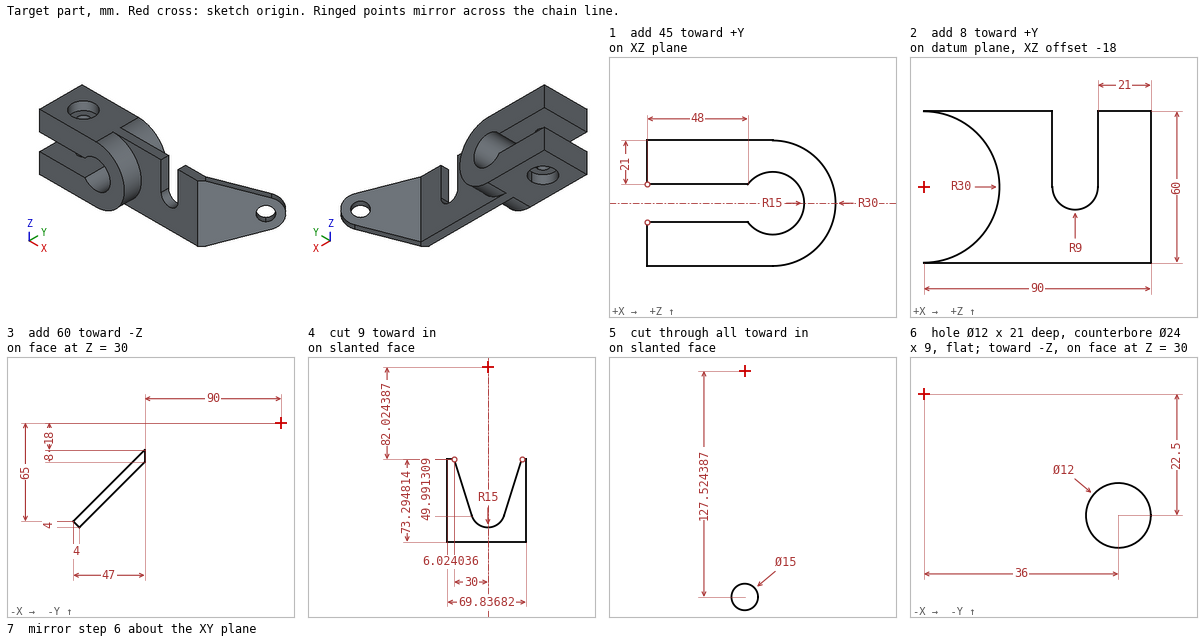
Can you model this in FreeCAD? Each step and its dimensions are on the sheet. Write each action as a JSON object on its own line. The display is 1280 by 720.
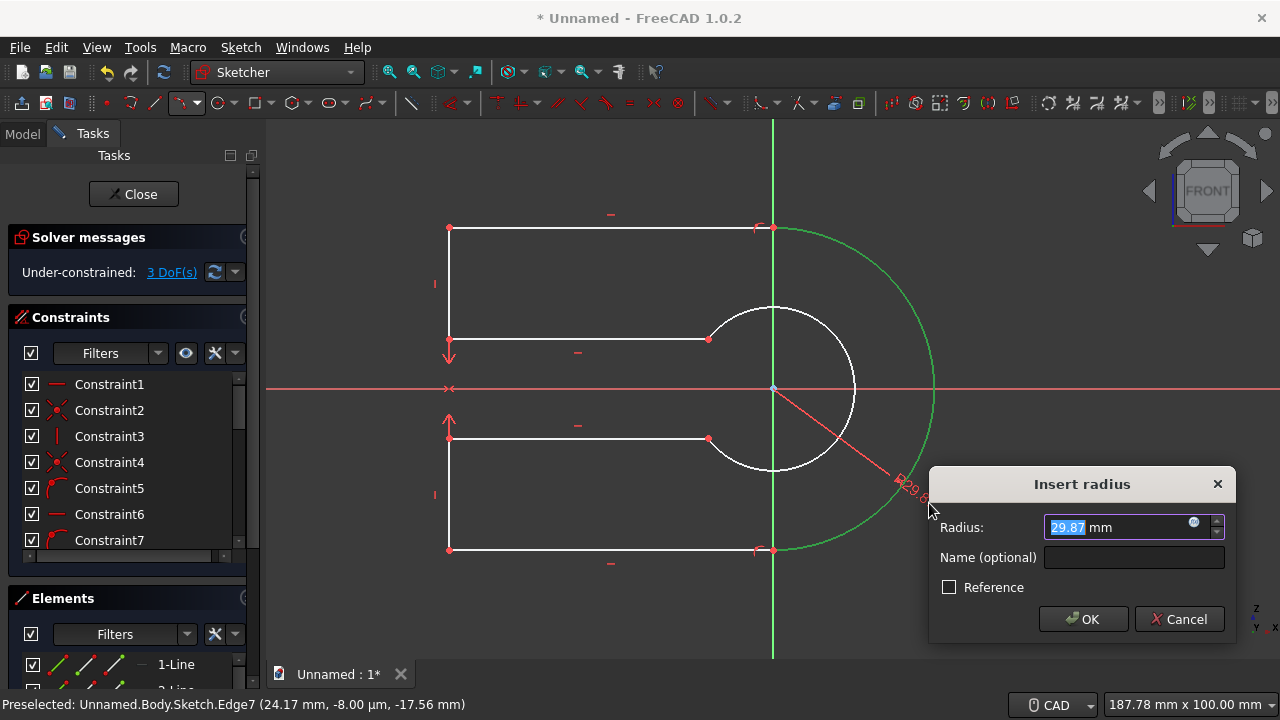
{"action": "type", "text": "30"}
{"action": "key", "text": "Return"}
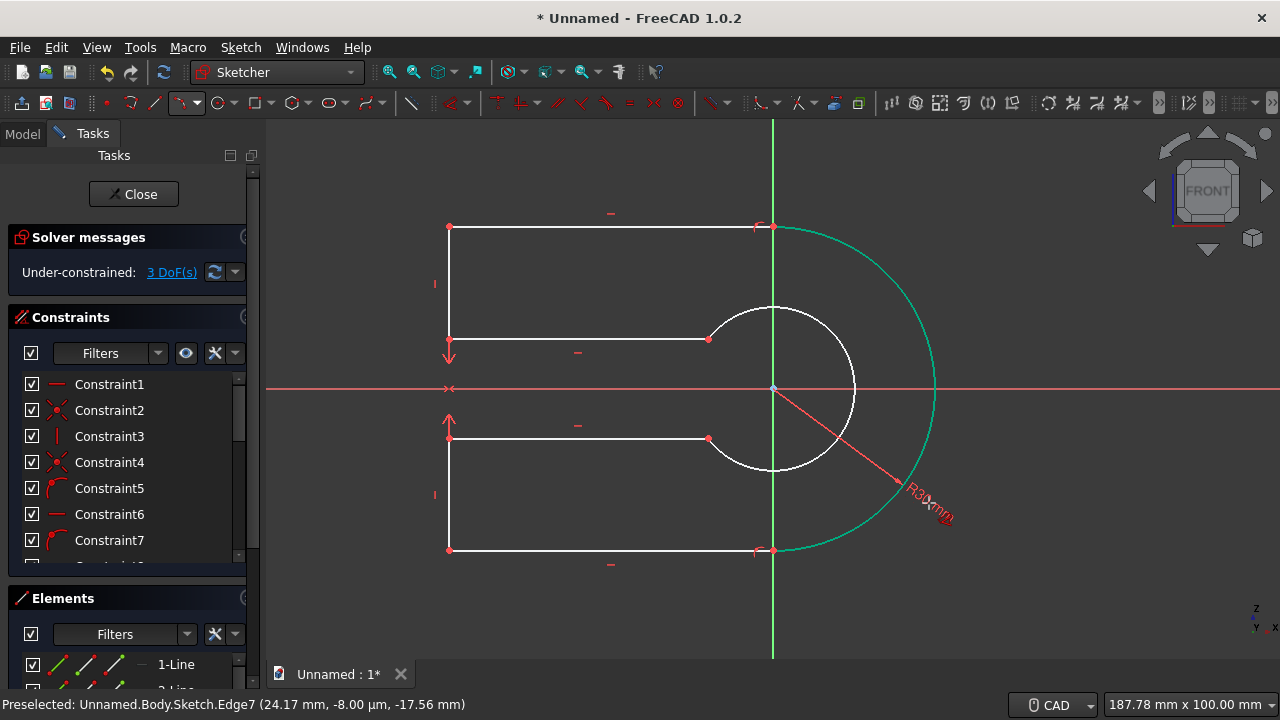
{"action": "left_click", "coordinate": [818, 458]}
{"action": "left_click", "coordinate": [835, 485]}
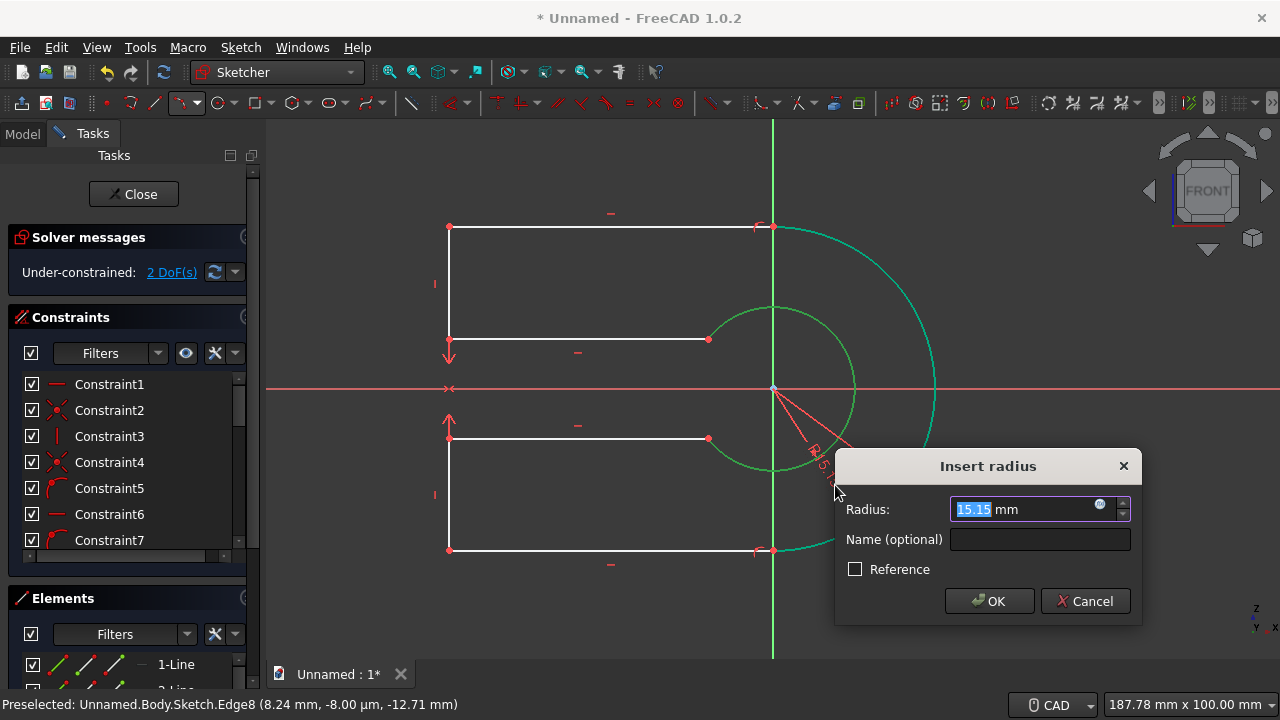
{"action": "type", "text": "15"}
{"action": "key", "text": "Return"}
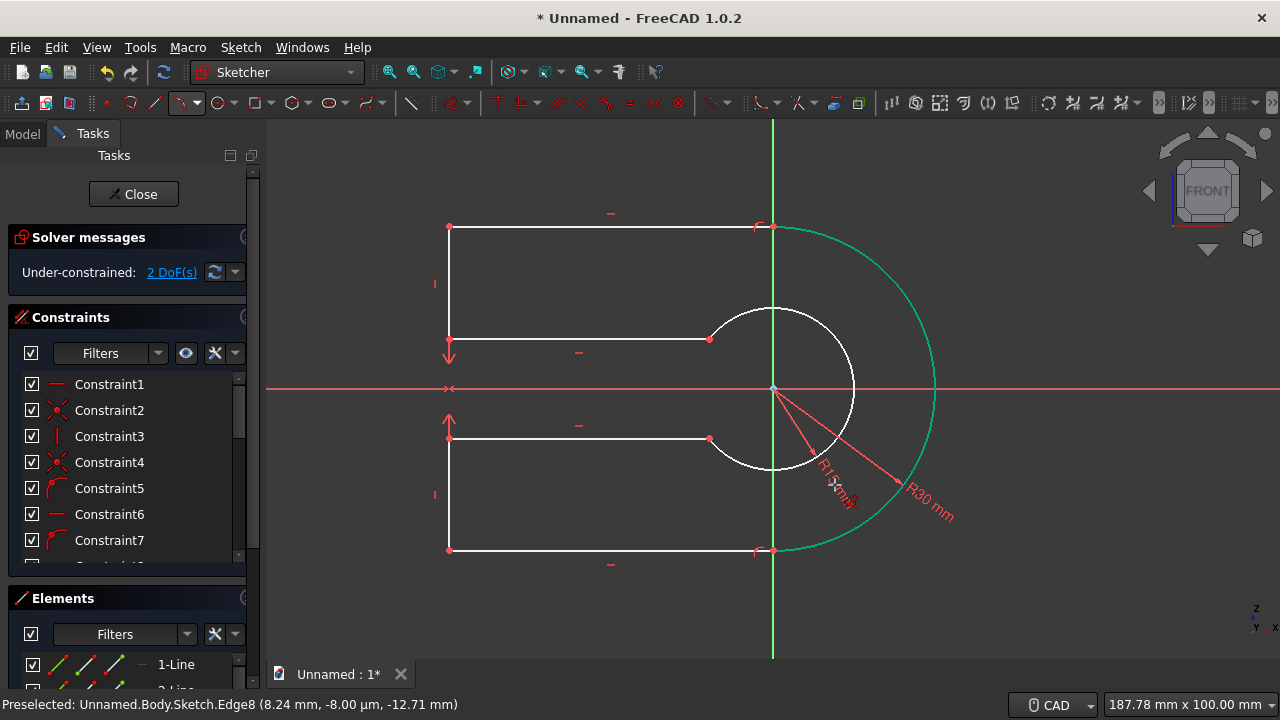
{"action": "left_click", "coordinate": [631, 339]}
{"action": "left_click", "coordinate": [579, 305]}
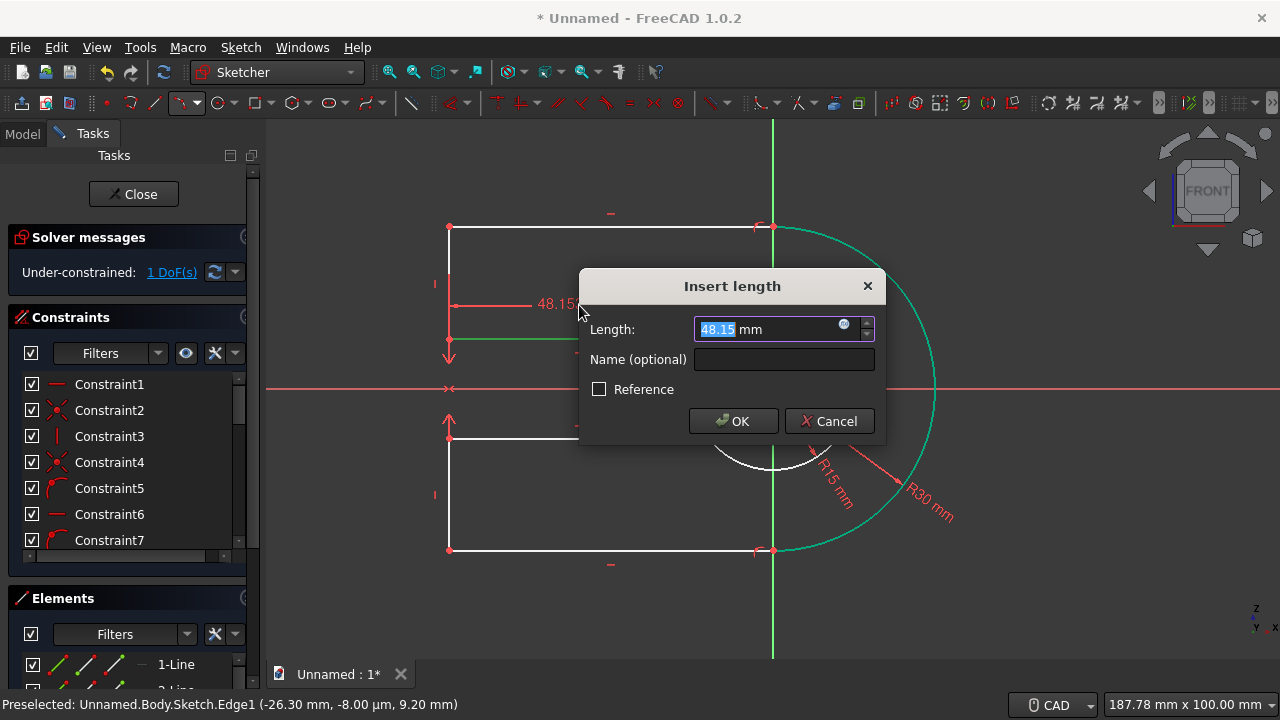
{"action": "type", "text": "48"}
{"action": "key", "text": "Return"}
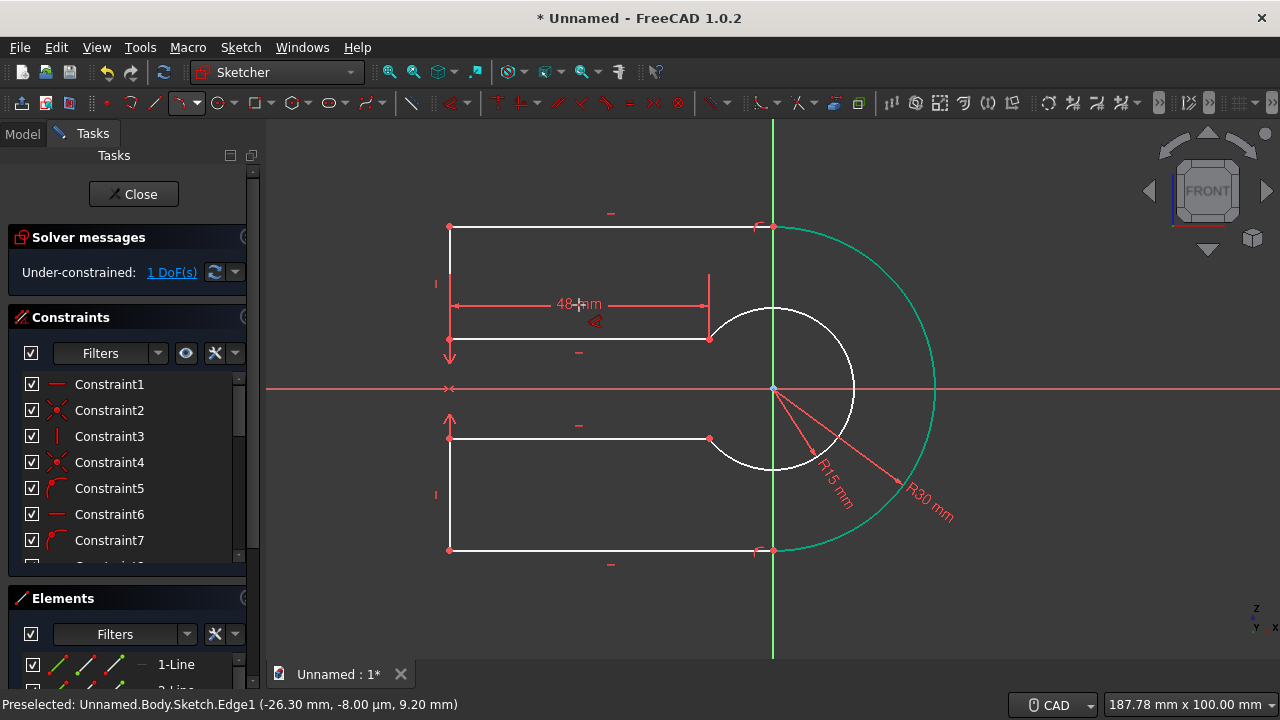
{"action": "left_click", "coordinate": [450, 306]}
{"action": "left_click", "coordinate": [416, 283]}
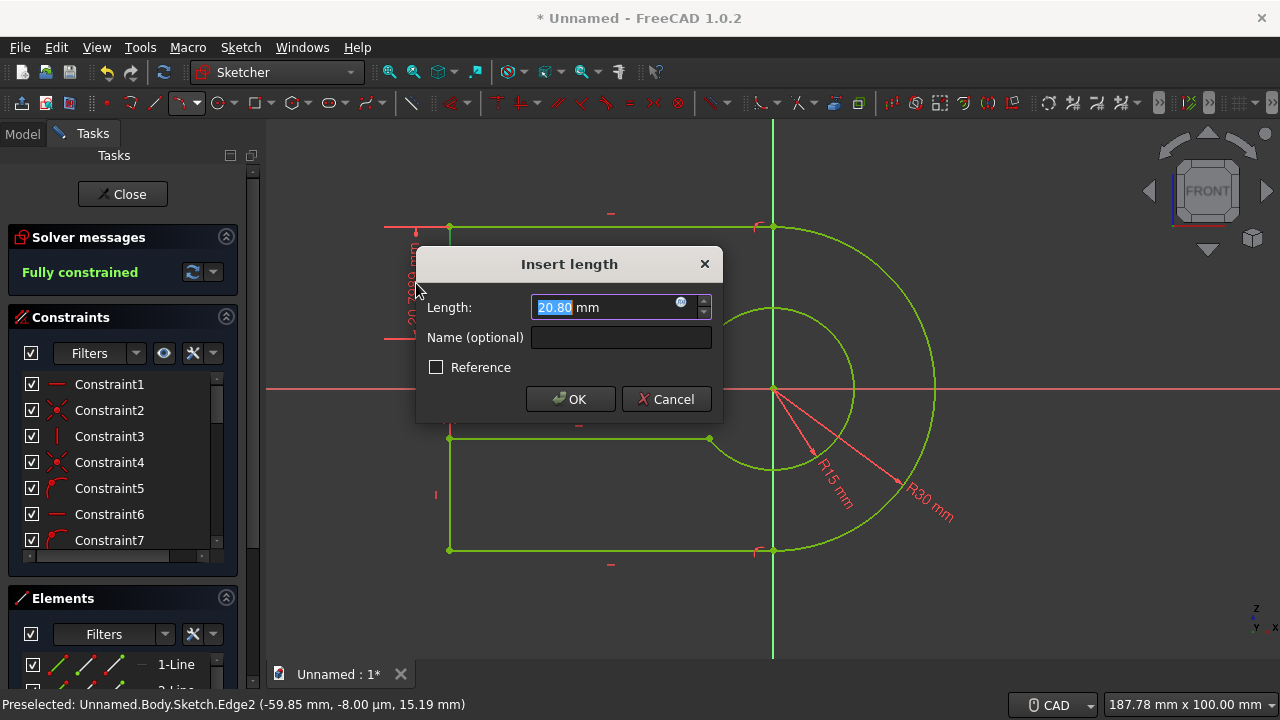
{"action": "type", "text": "21"}
{"action": "key", "text": "Return"}
{"action": "key", "text": "Escape"}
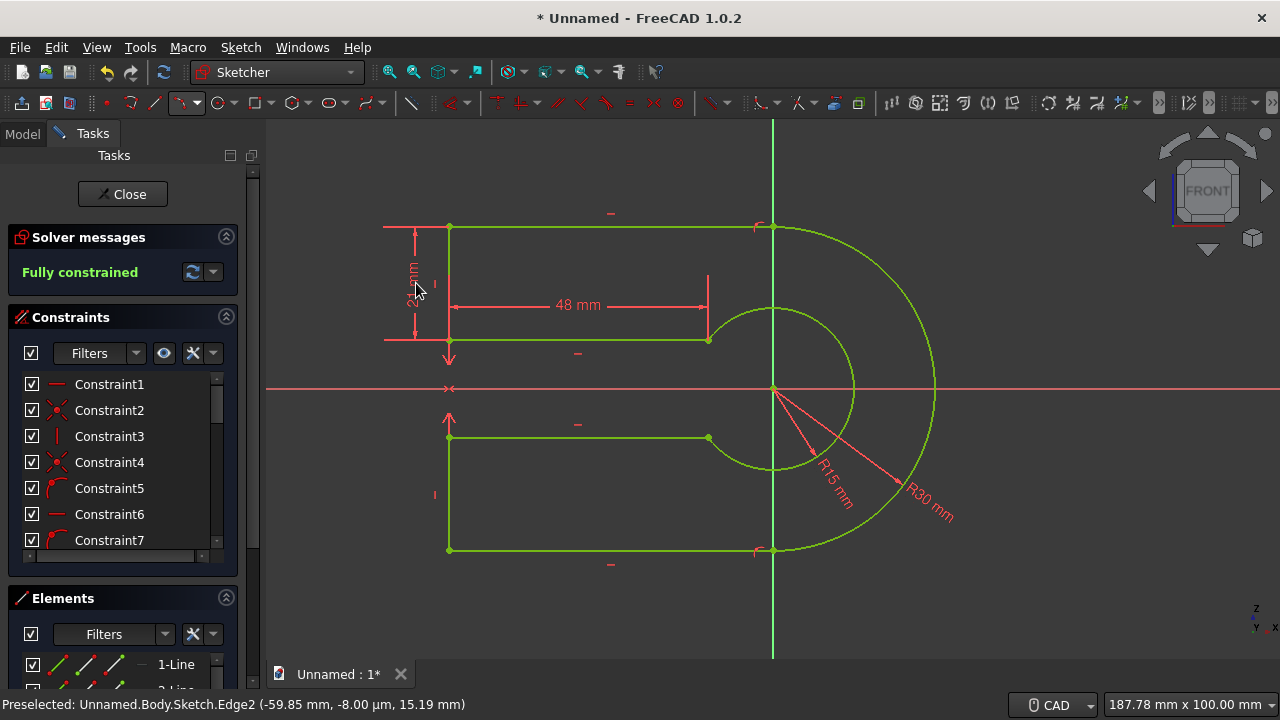
{"action": "left_click", "coordinate": [123, 194]}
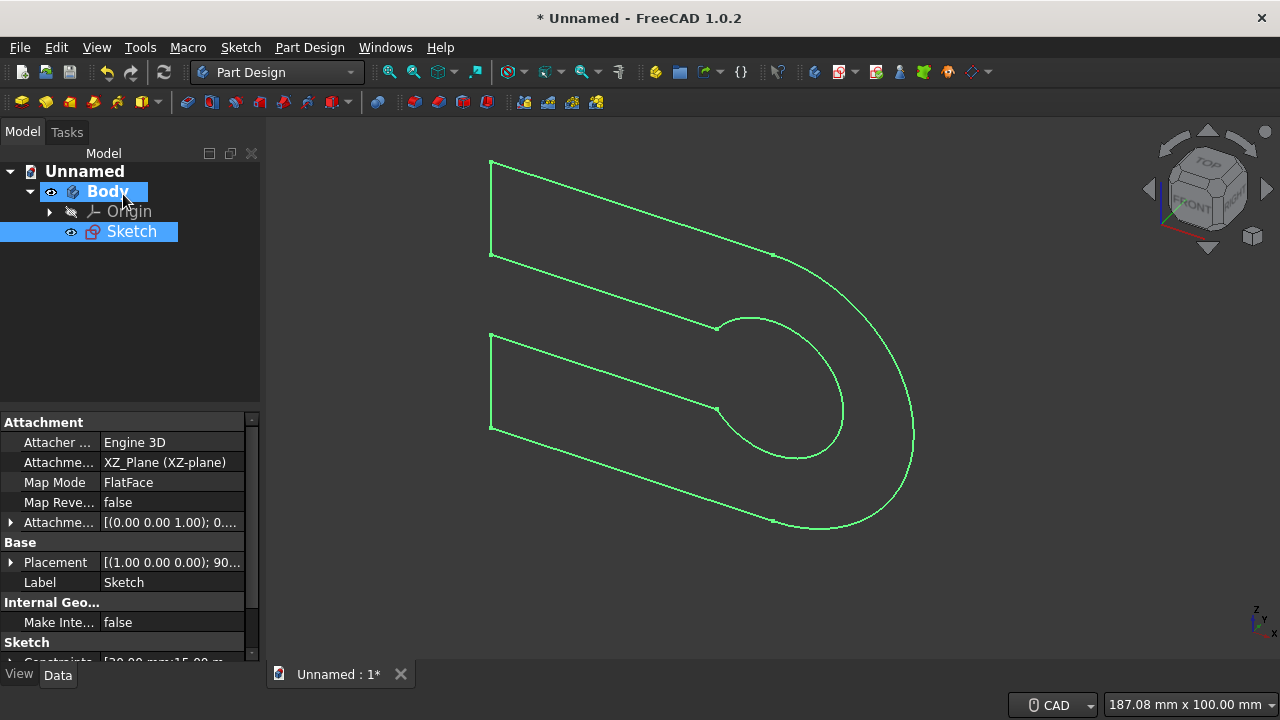
{"action": "left_click", "coordinate": [22, 102]}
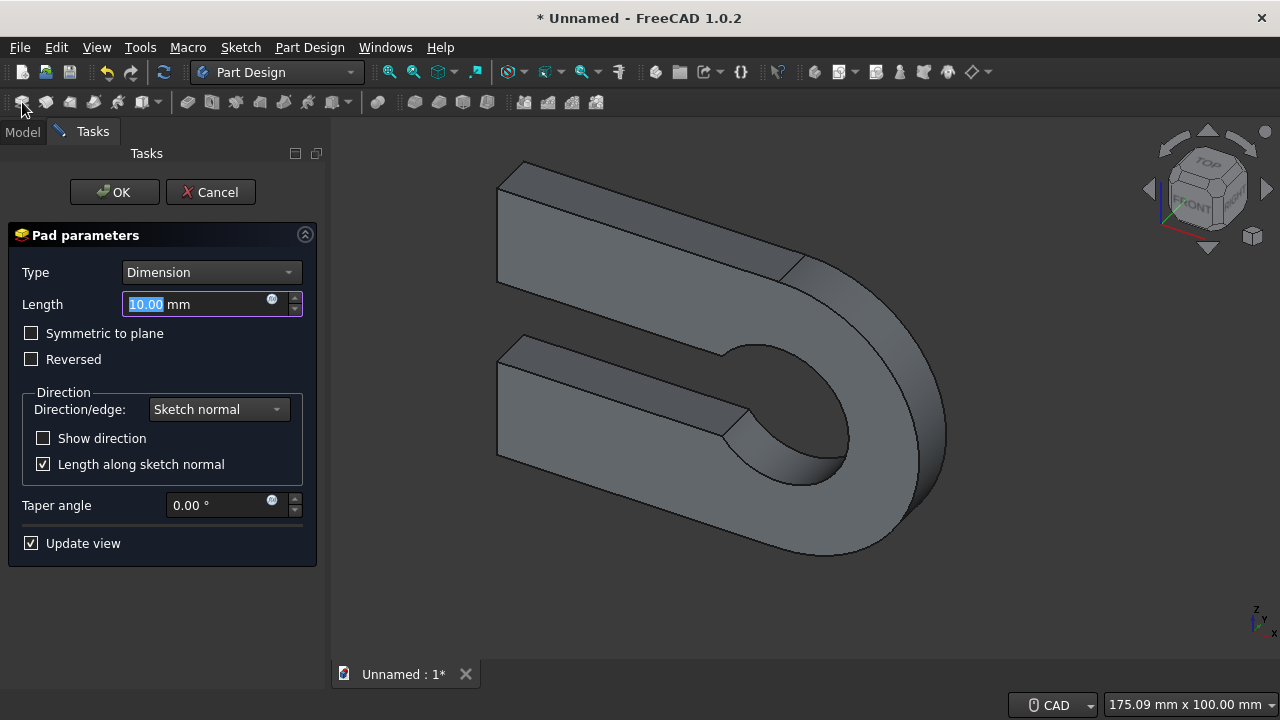
{"action": "type", "text": "45"}
{"action": "key", "text": "Tab"}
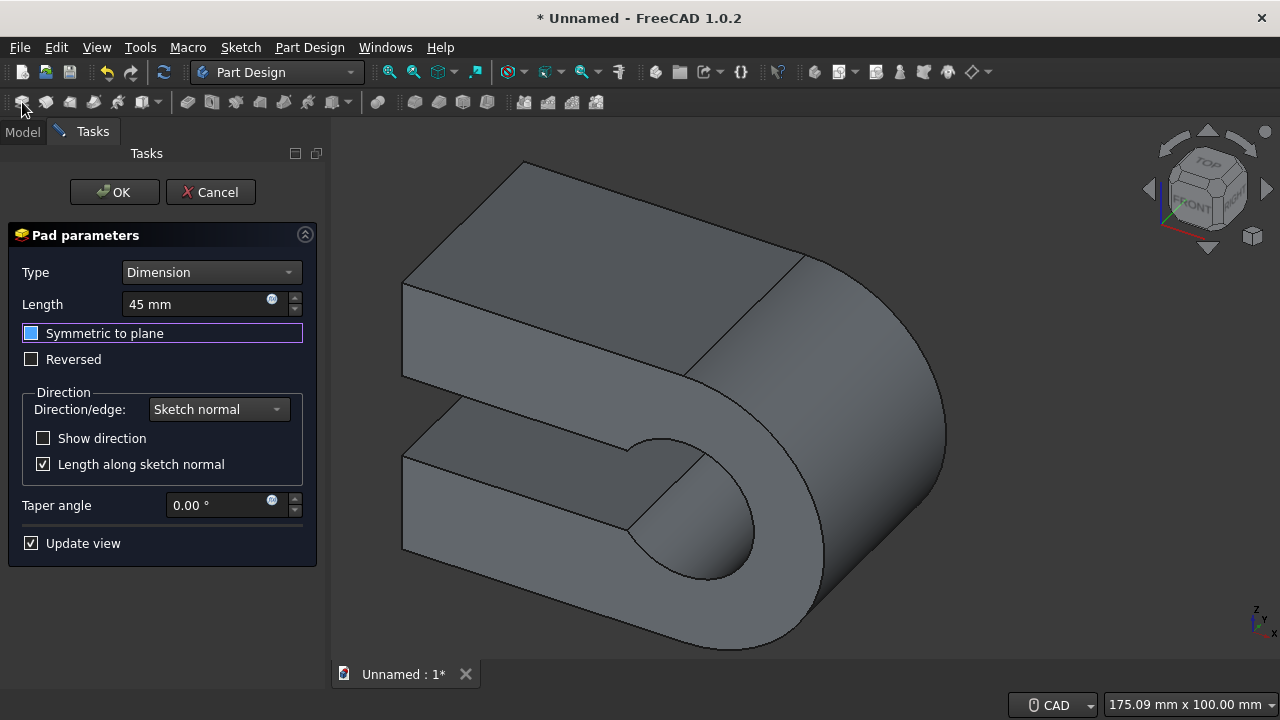
{"action": "left_click", "coordinate": [30, 359]}